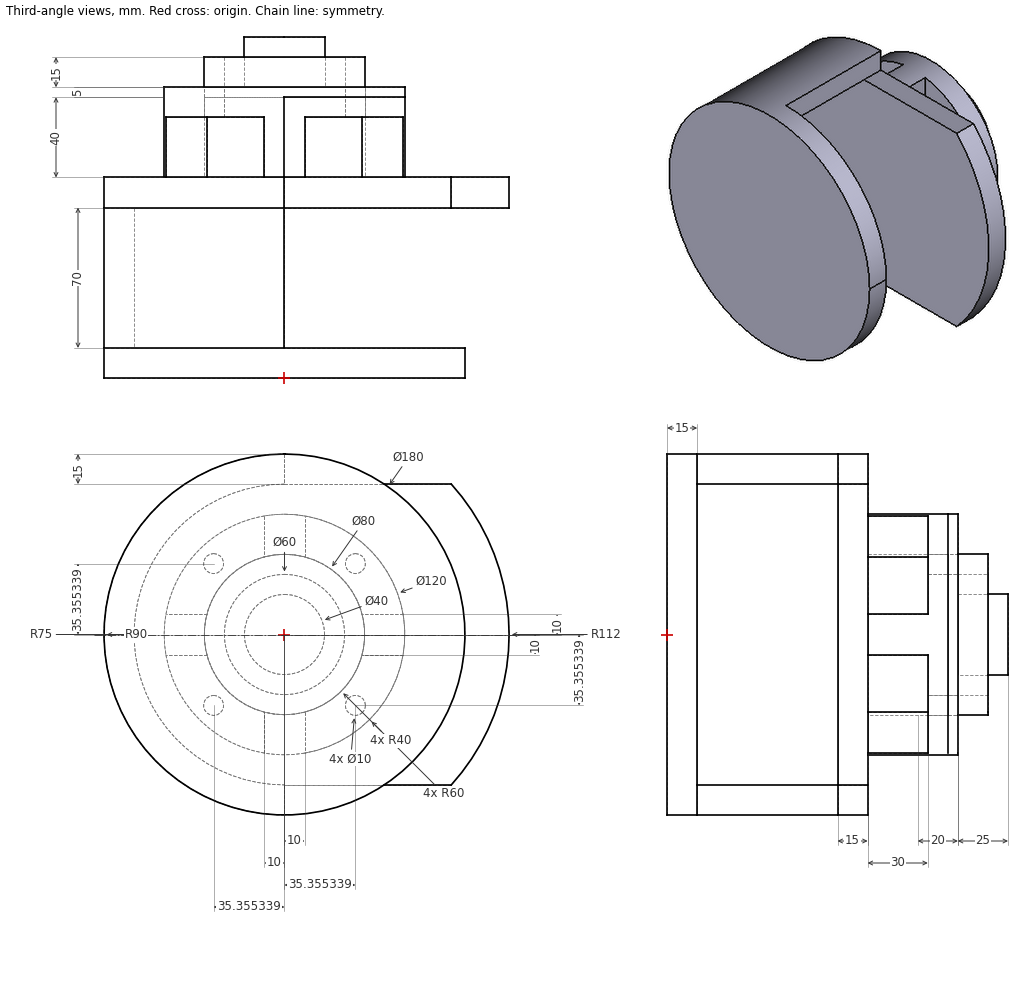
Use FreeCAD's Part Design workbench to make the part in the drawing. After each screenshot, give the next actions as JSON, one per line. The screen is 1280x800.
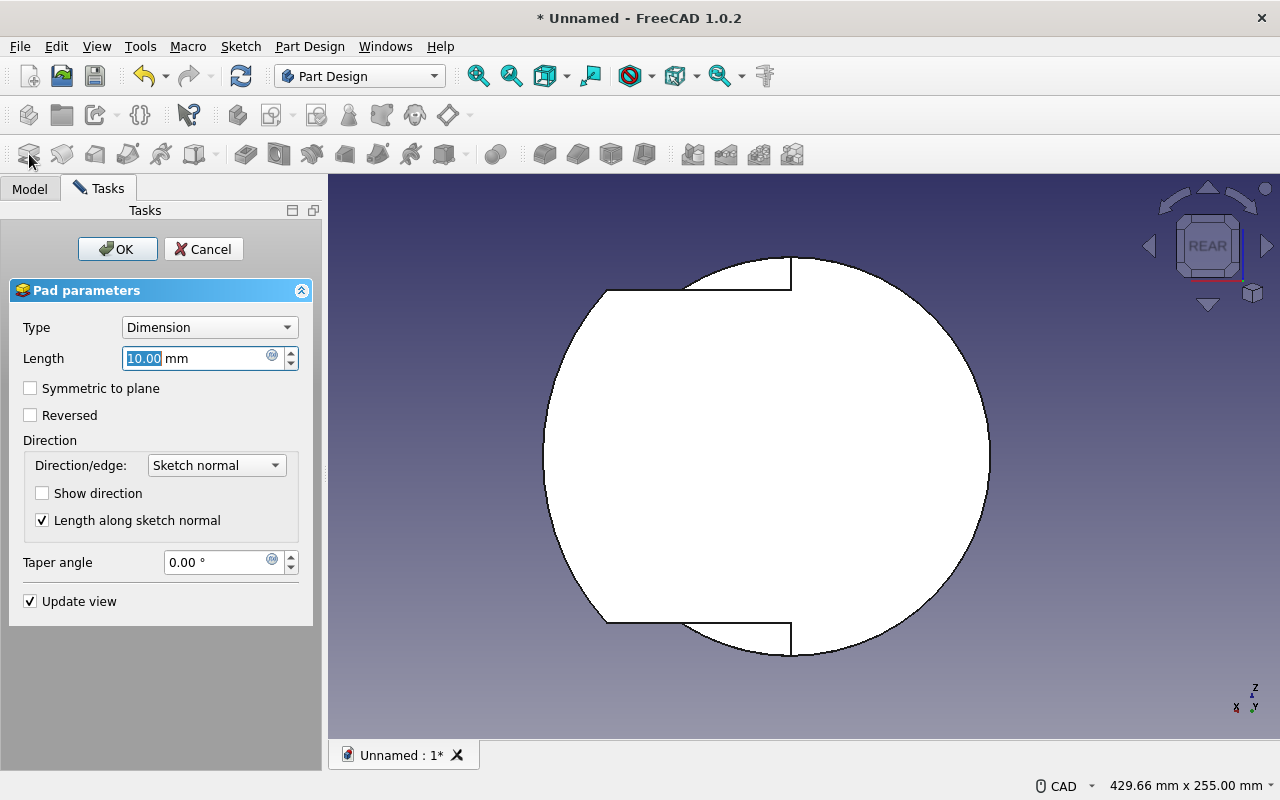
{"action": "type", "text": "15"}
{"action": "key", "text": "Tab"}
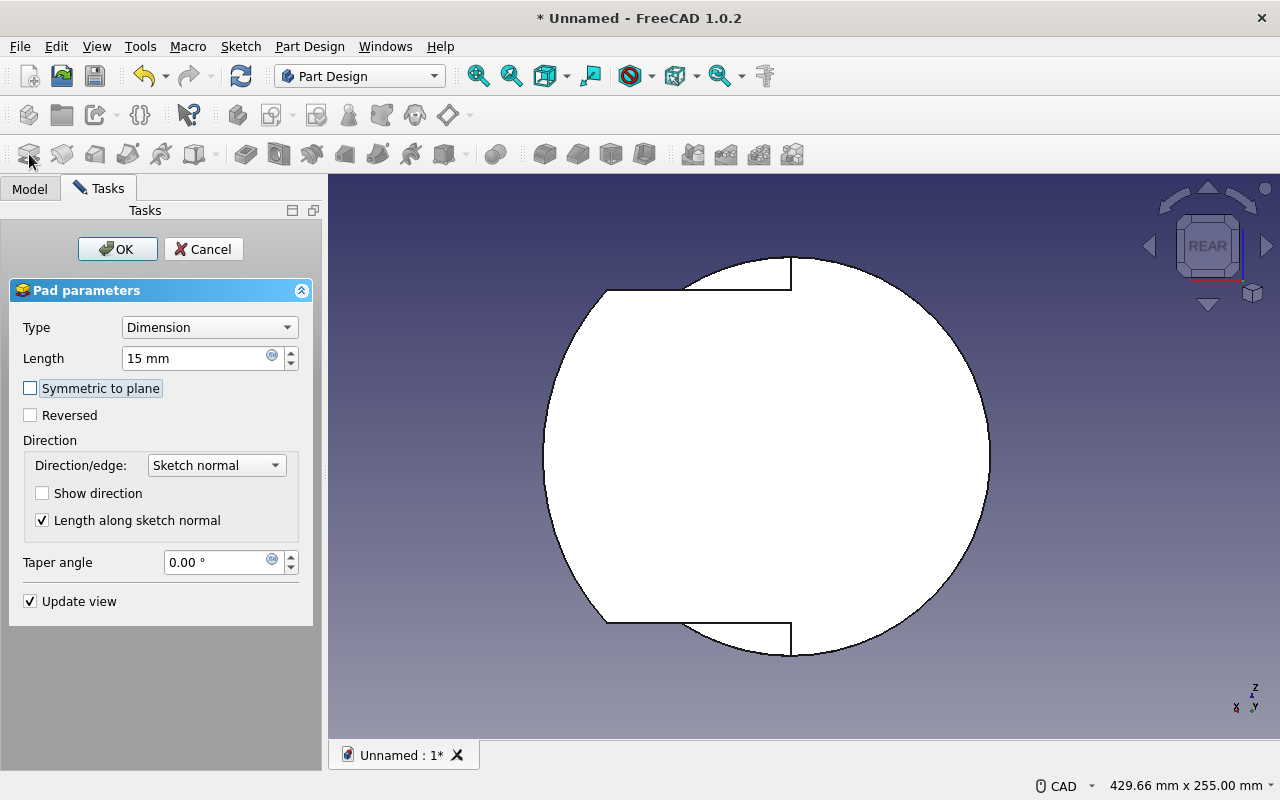
{"action": "left_click", "coordinate": [118, 249]}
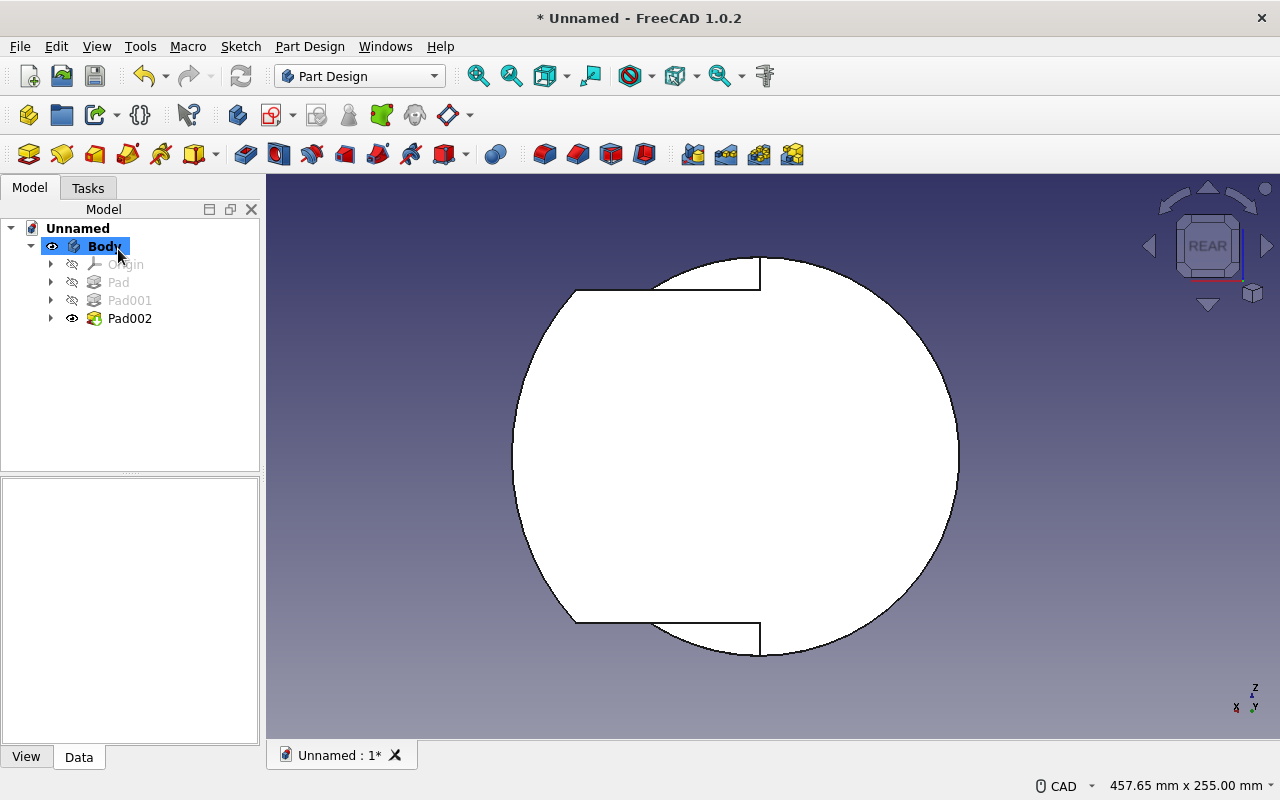
{"action": "left_click", "coordinate": [736, 455]}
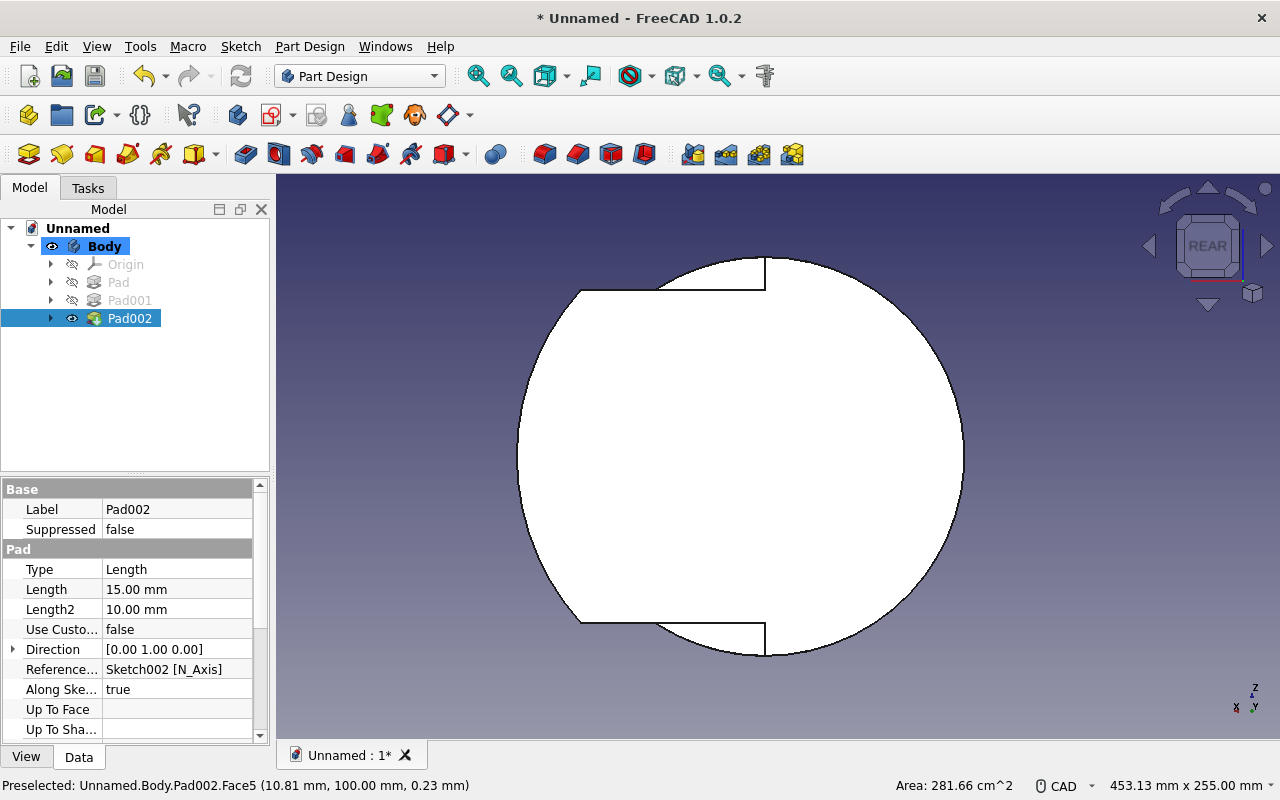
{"action": "left_click", "coordinate": [270, 116]}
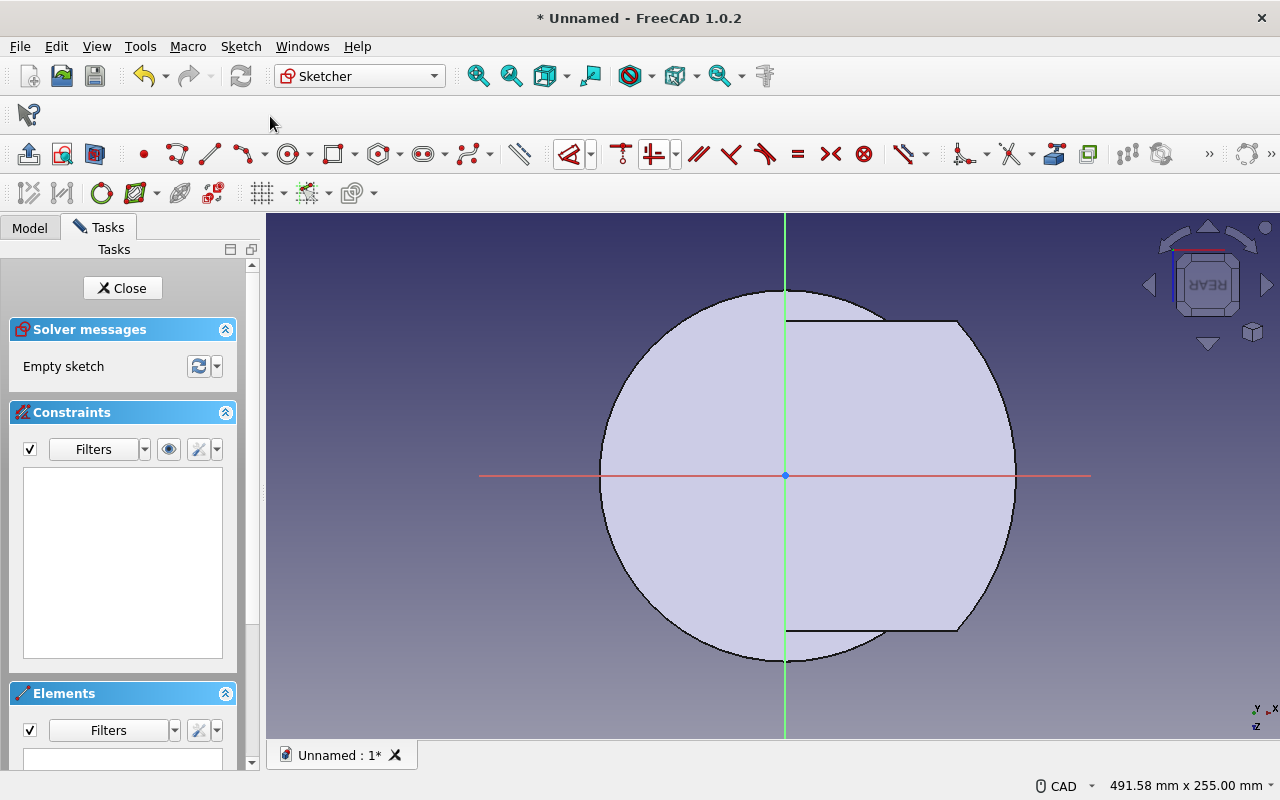
{"action": "key", "text": "g c"}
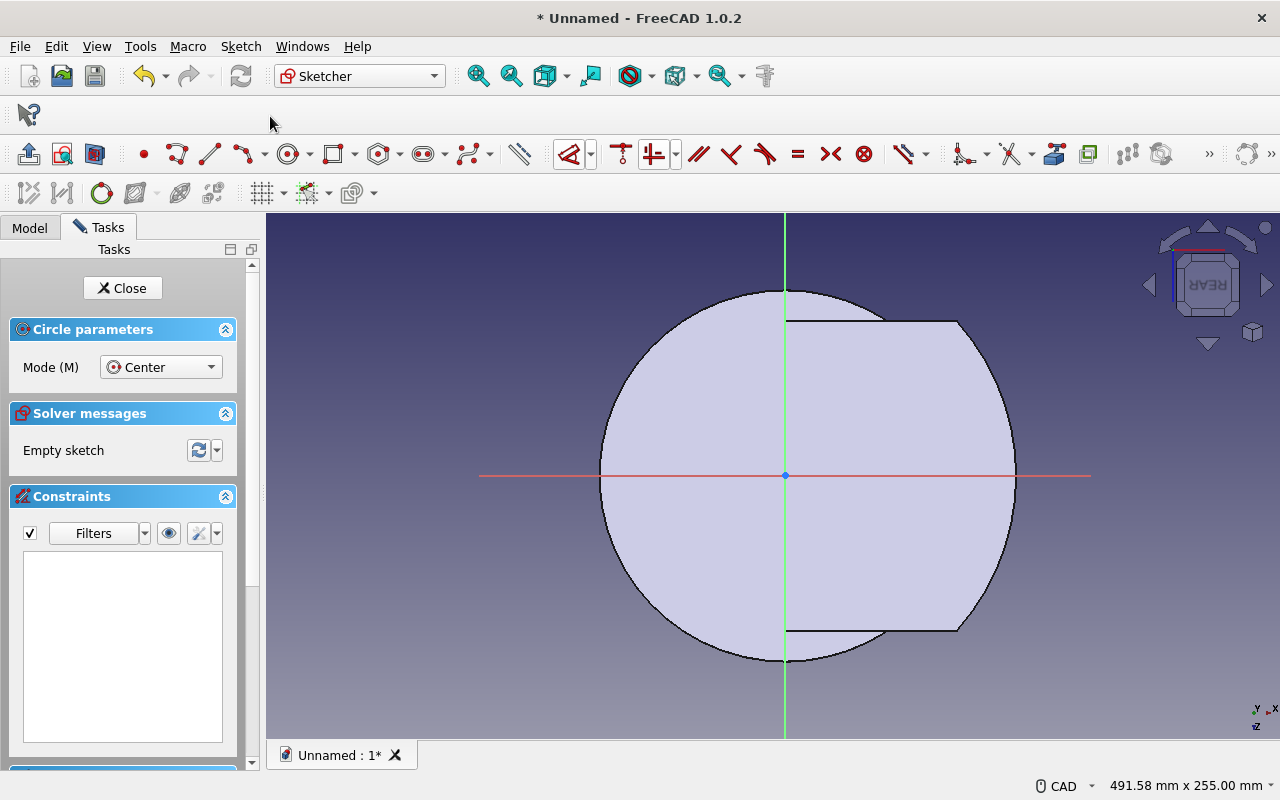
{"action": "left_click", "coordinate": [785, 476]}
{"action": "left_click", "coordinate": [873, 388]}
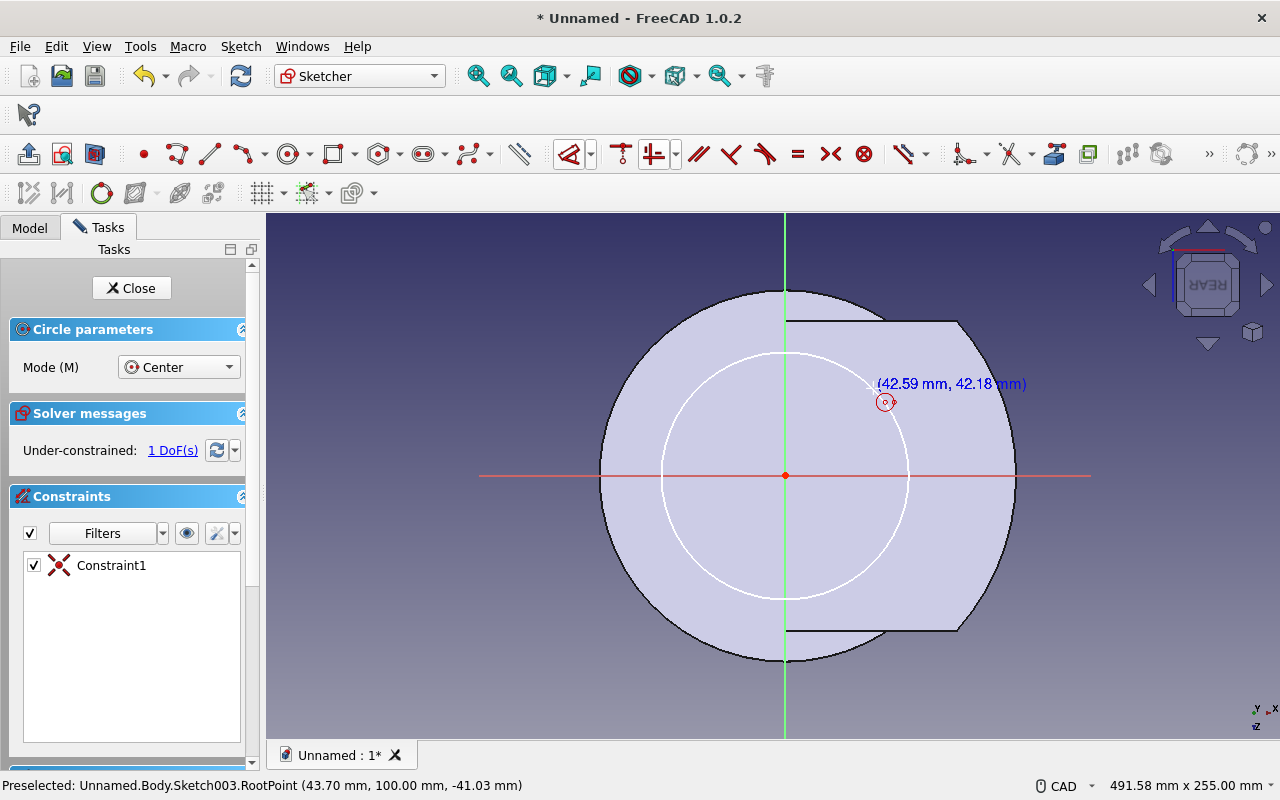
{"action": "left_click", "coordinate": [785, 476]}
{"action": "left_click", "coordinate": [843, 418]}
{"action": "key", "text": "Escape"}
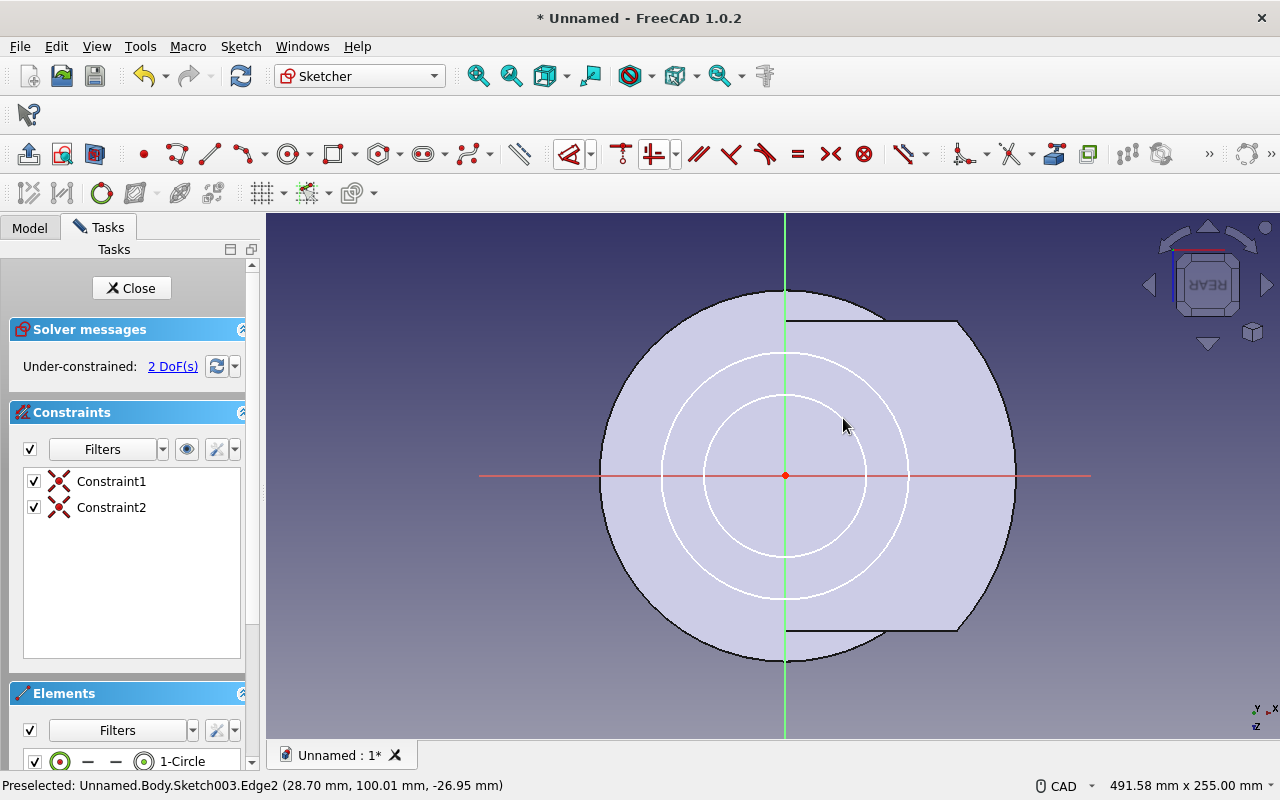
{"action": "left_click", "coordinate": [872, 388]}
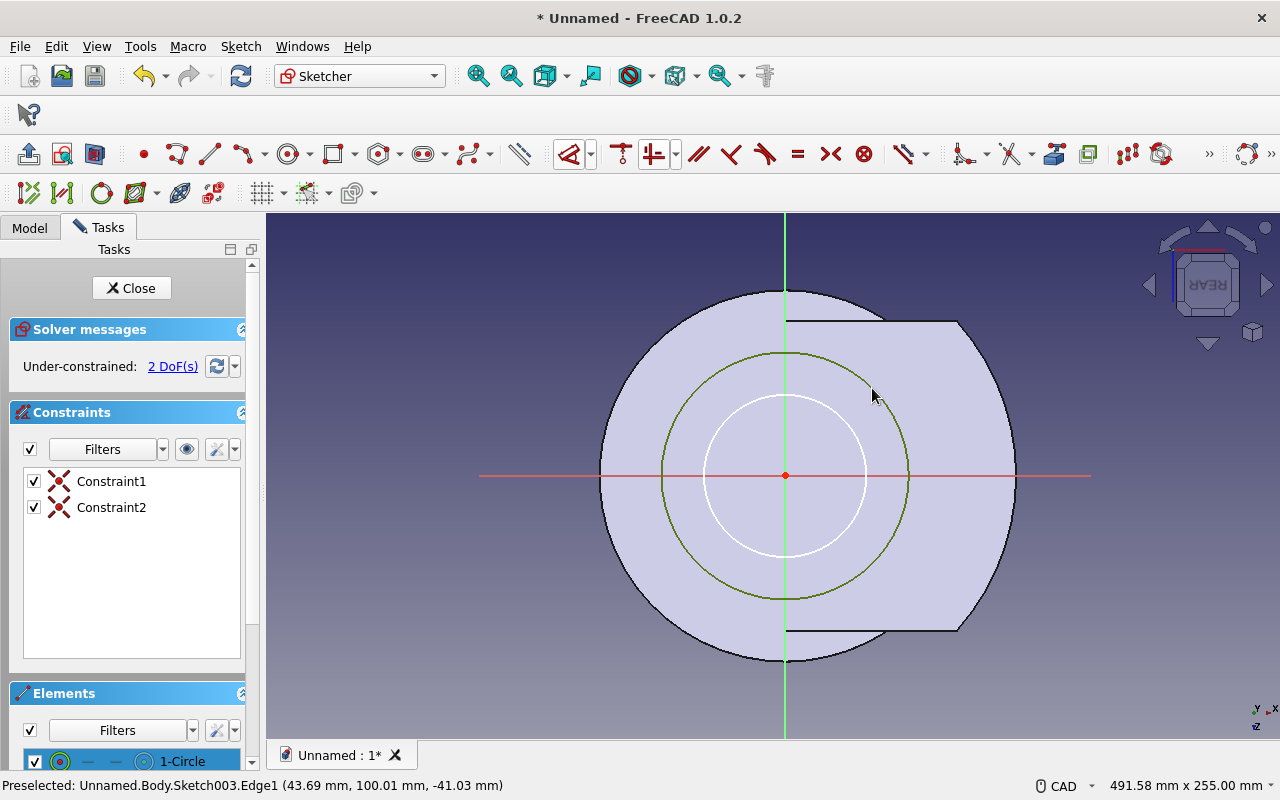
{"action": "left_click", "coordinate": [590, 154]}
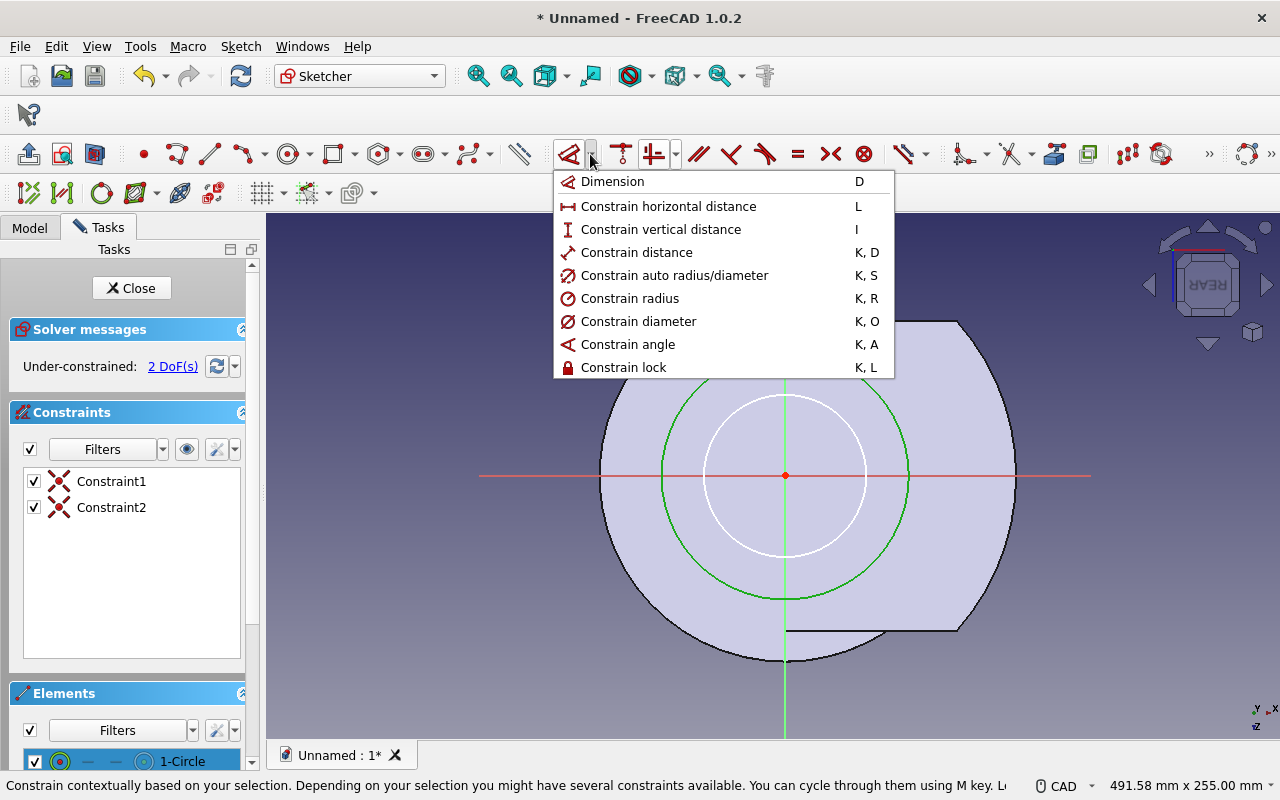
{"action": "left_click", "coordinate": [724, 322]}